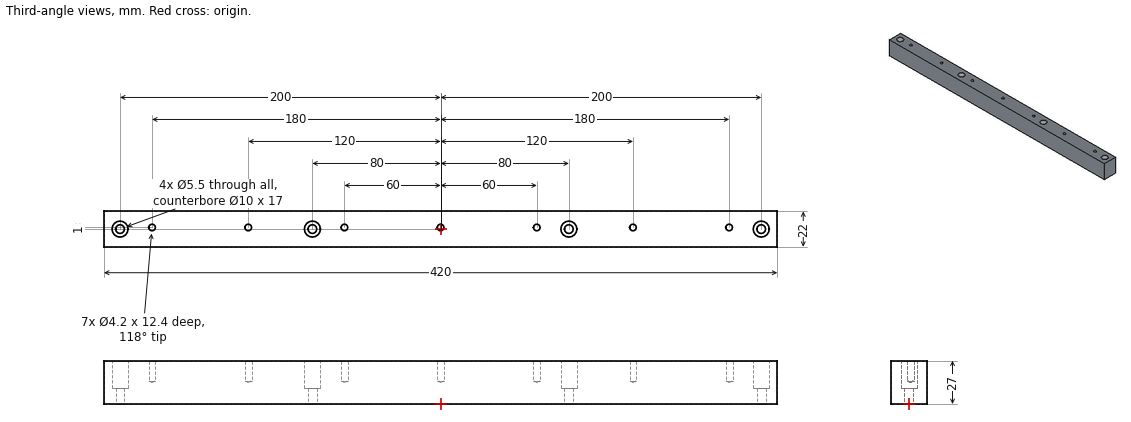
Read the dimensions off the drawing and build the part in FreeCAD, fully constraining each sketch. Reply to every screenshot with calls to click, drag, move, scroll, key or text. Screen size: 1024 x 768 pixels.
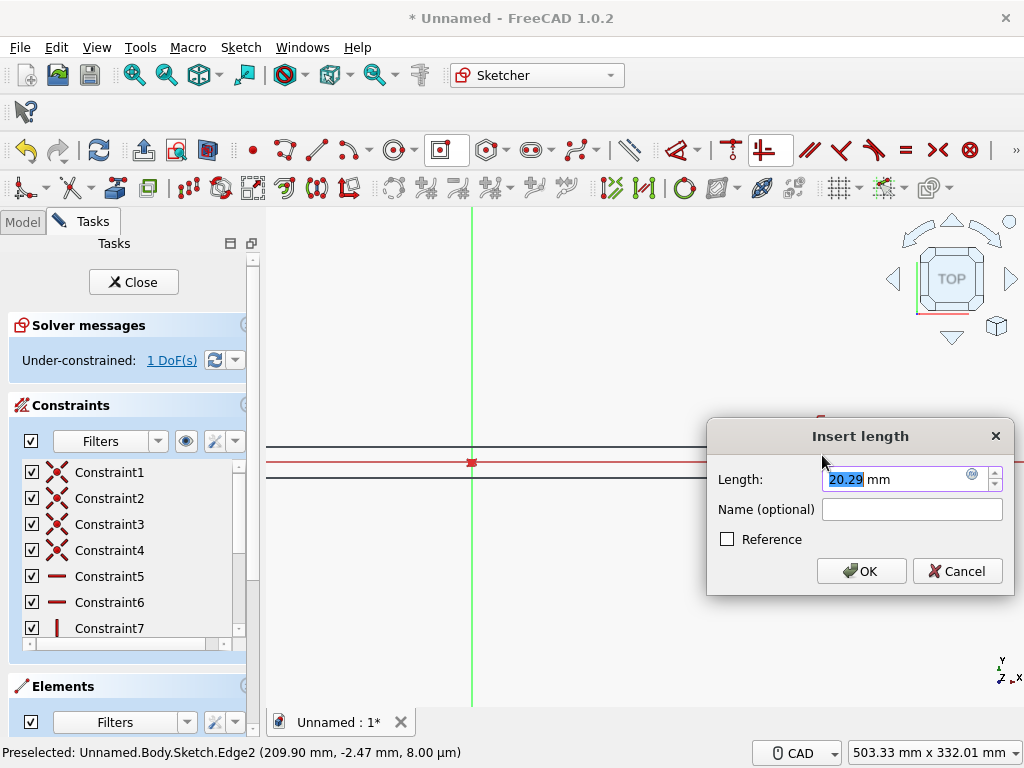
text(22)
key(Return)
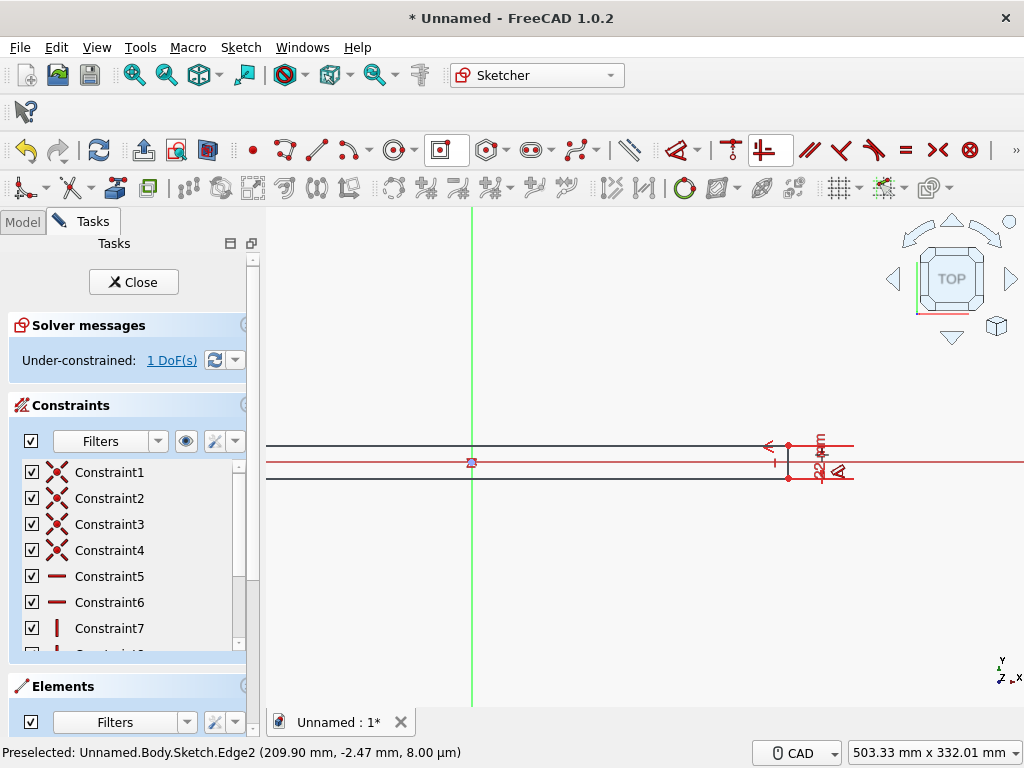
click(345, 479)
click(541, 513)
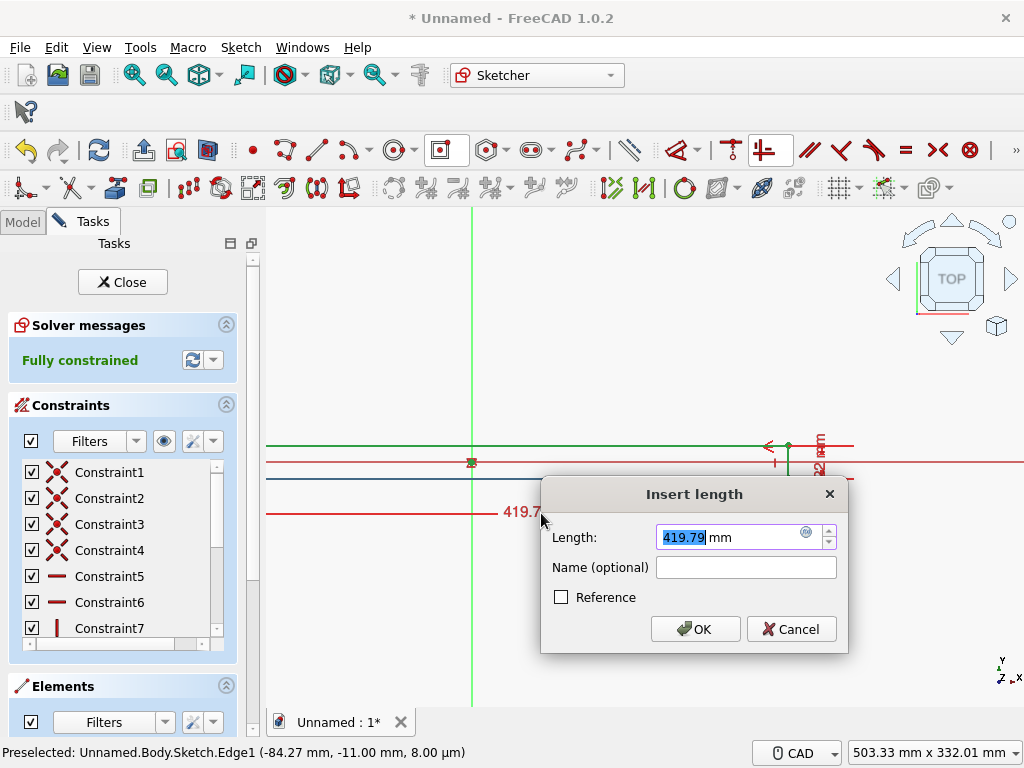
text(420)
key(Return)
key(Escape)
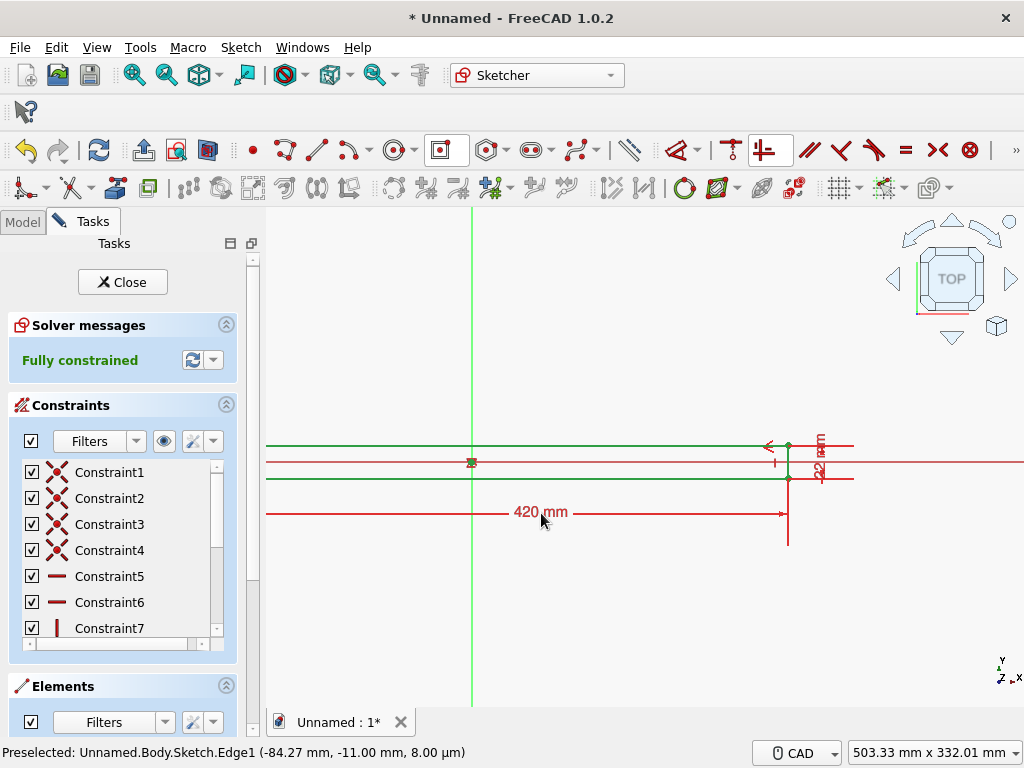
click(123, 282)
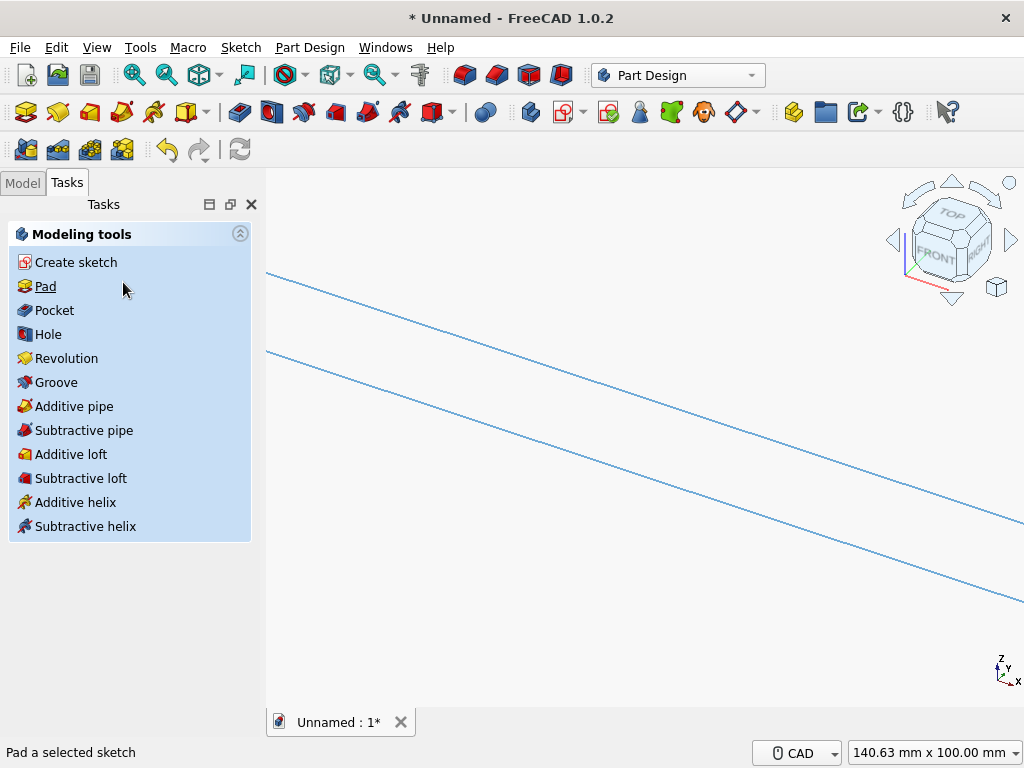
click(26, 112)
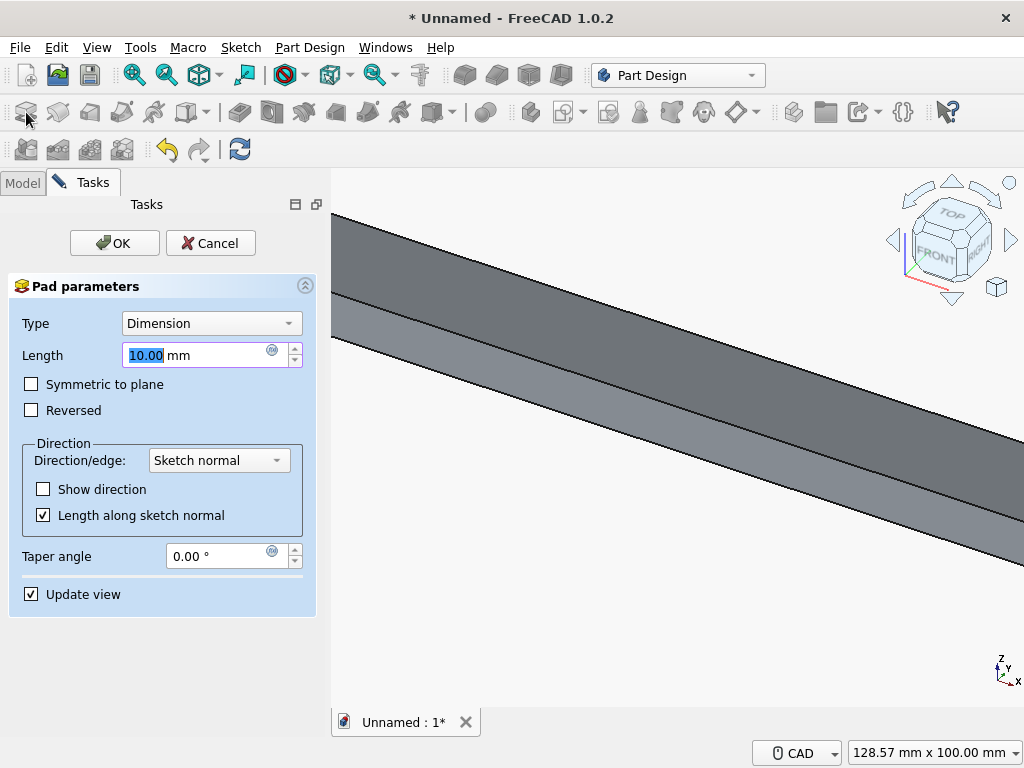
text(27)
key(Tab)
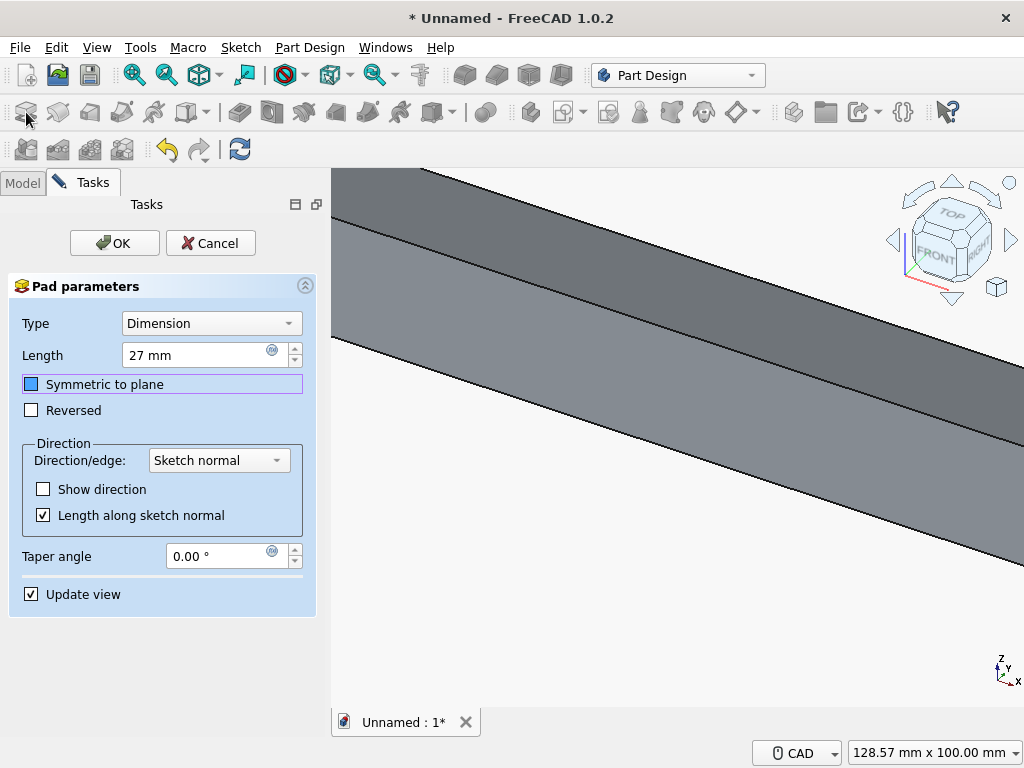
click(115, 243)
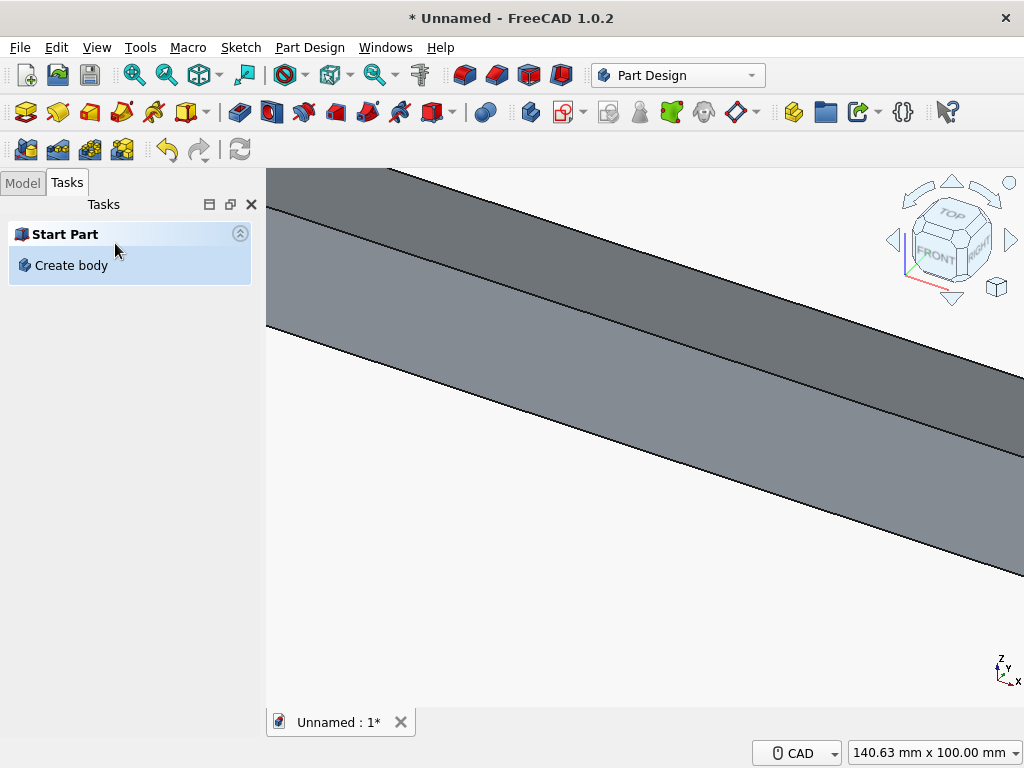
key(v)
key(f)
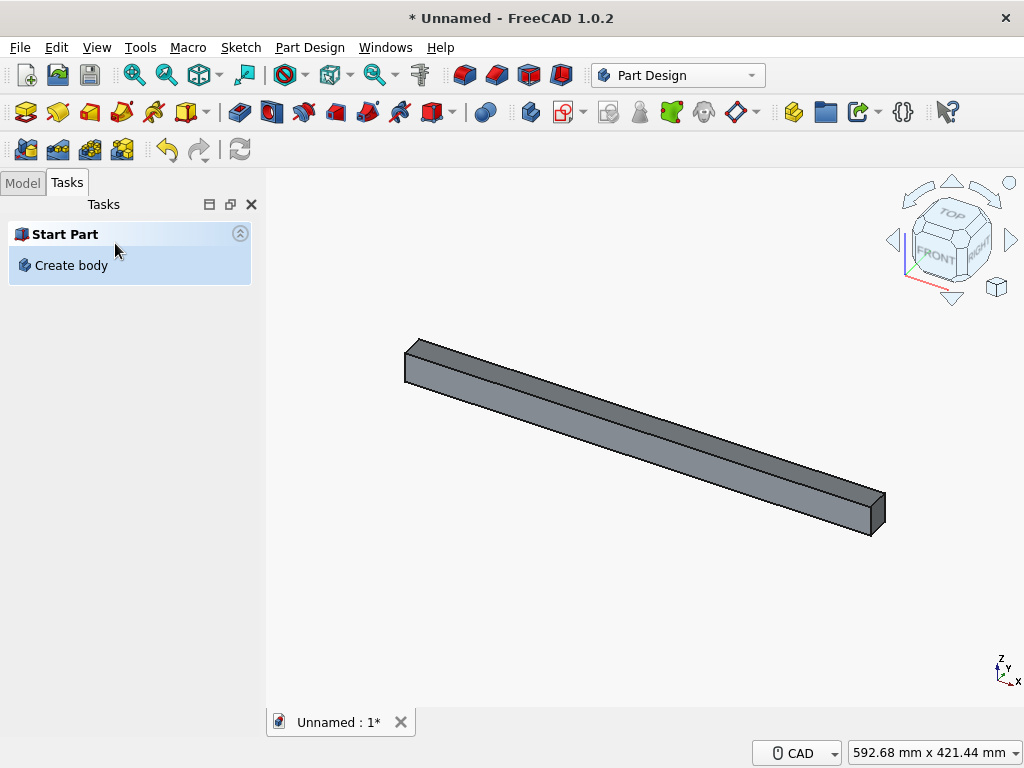
click(844, 488)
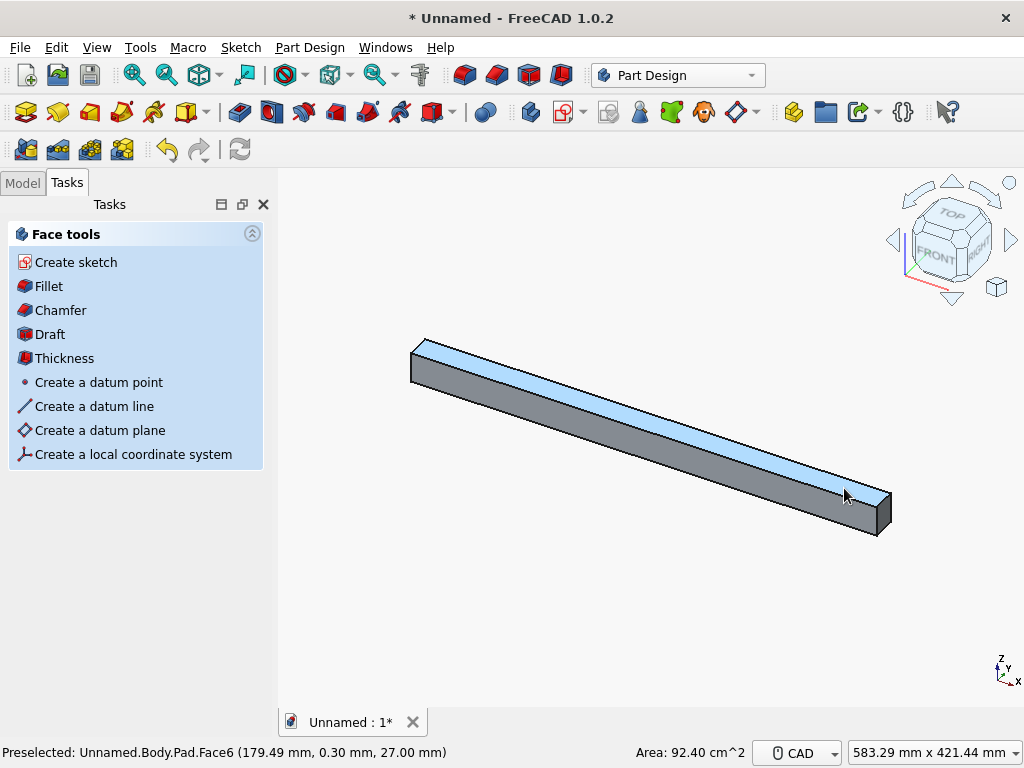
click(564, 112)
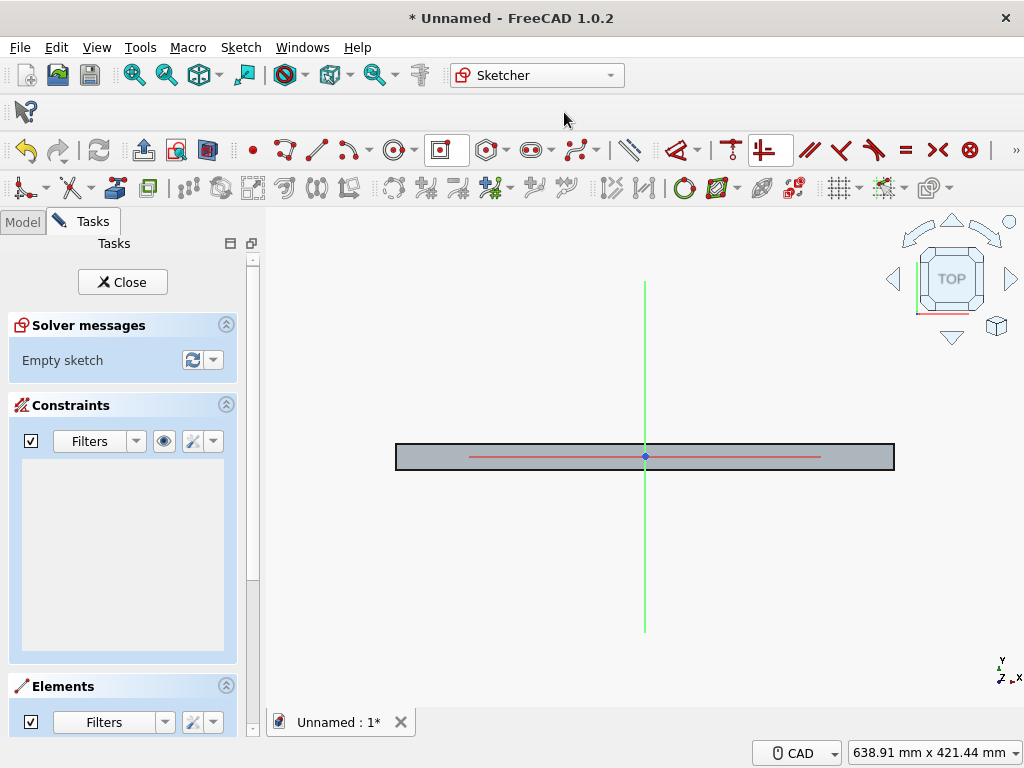
scroll(294, 462, down, 1)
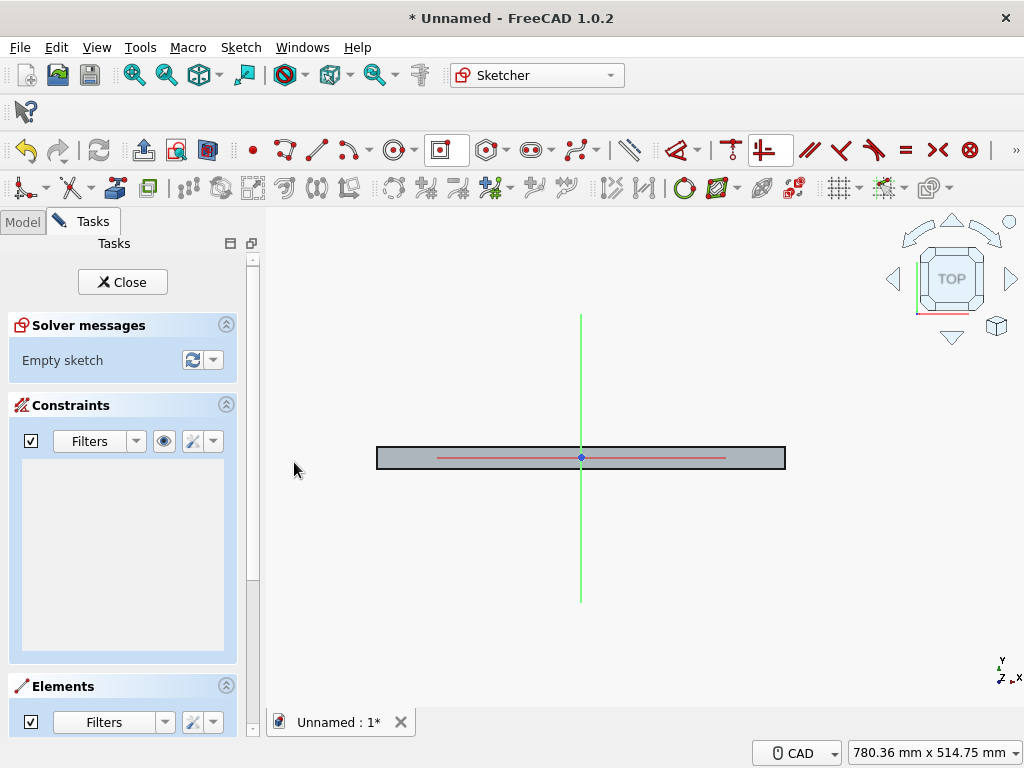
key(g)
key(c)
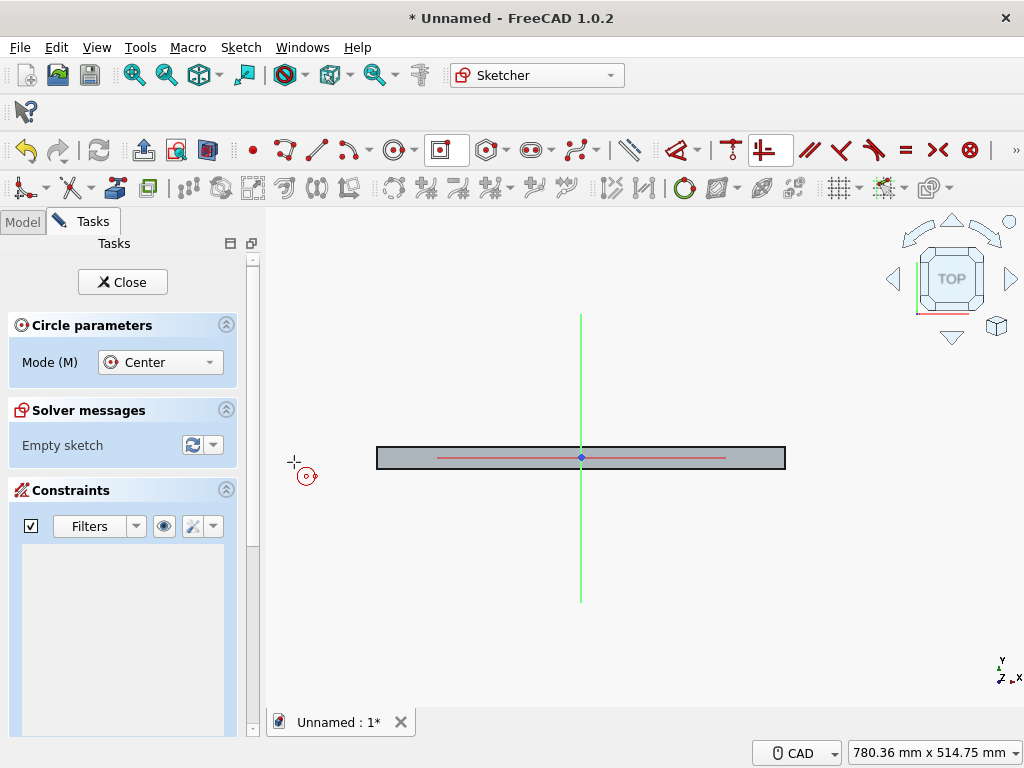
scroll(407, 457, up, 14)